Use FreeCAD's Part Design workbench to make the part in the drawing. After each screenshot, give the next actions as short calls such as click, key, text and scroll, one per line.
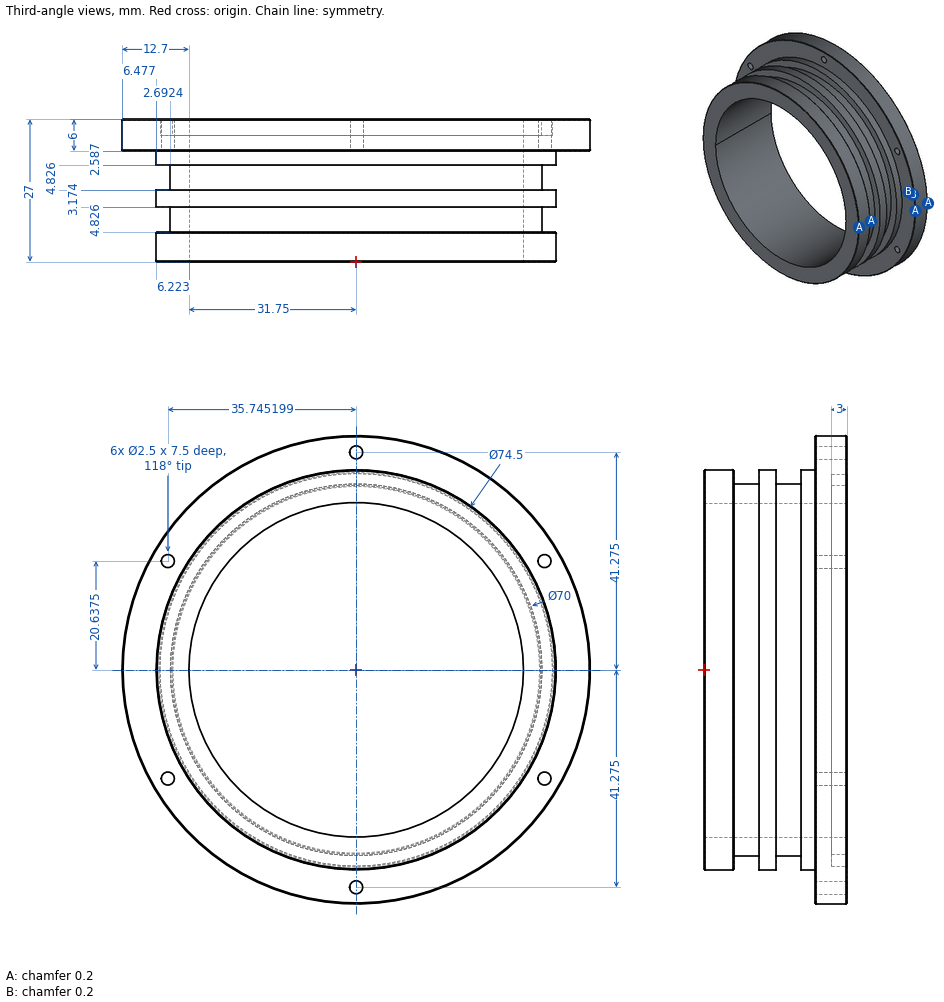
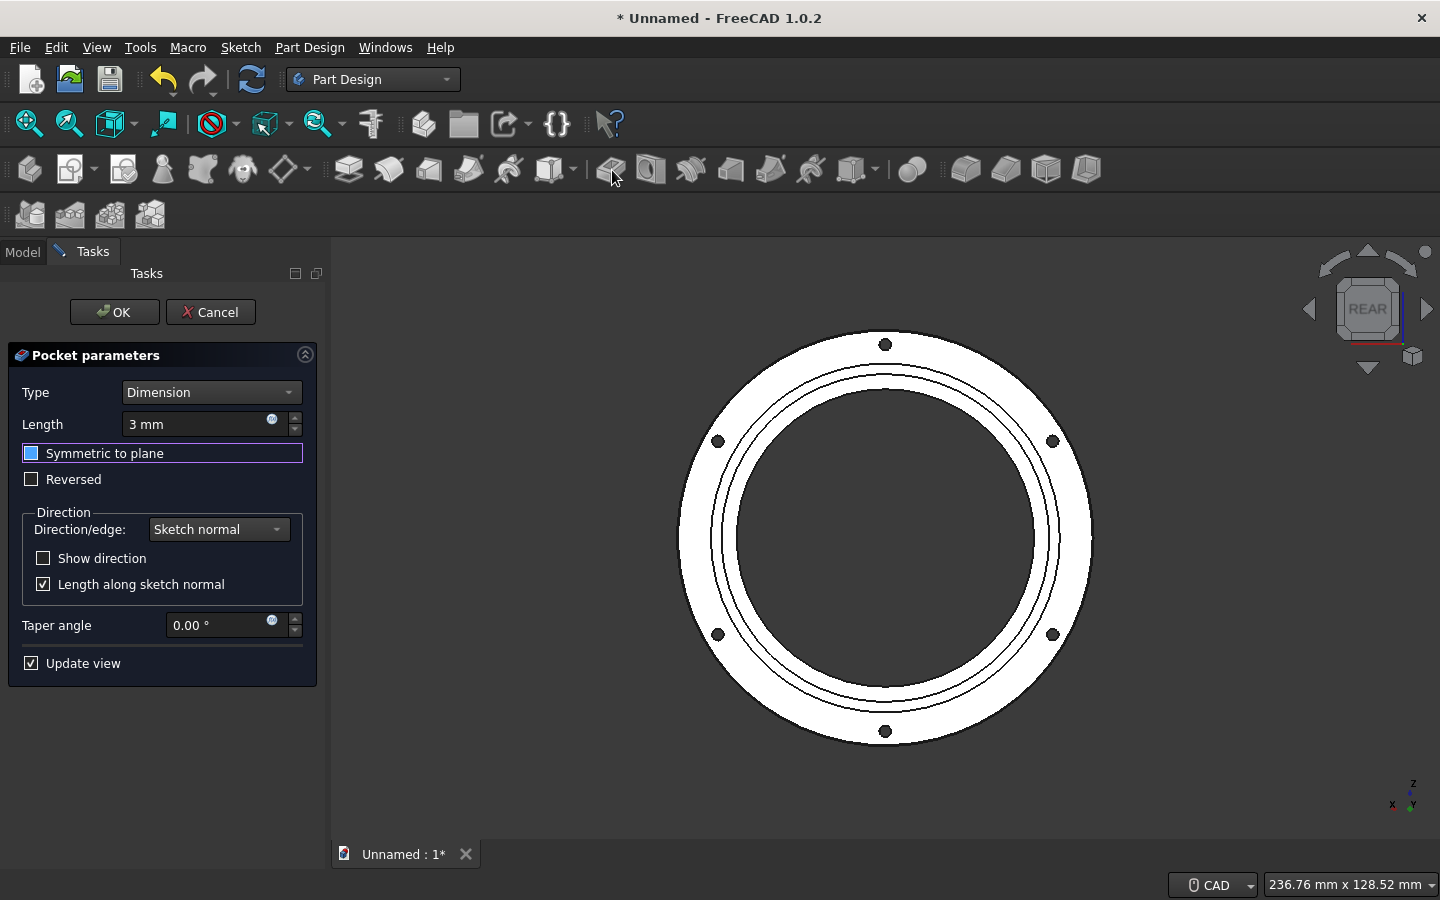
click(115, 312)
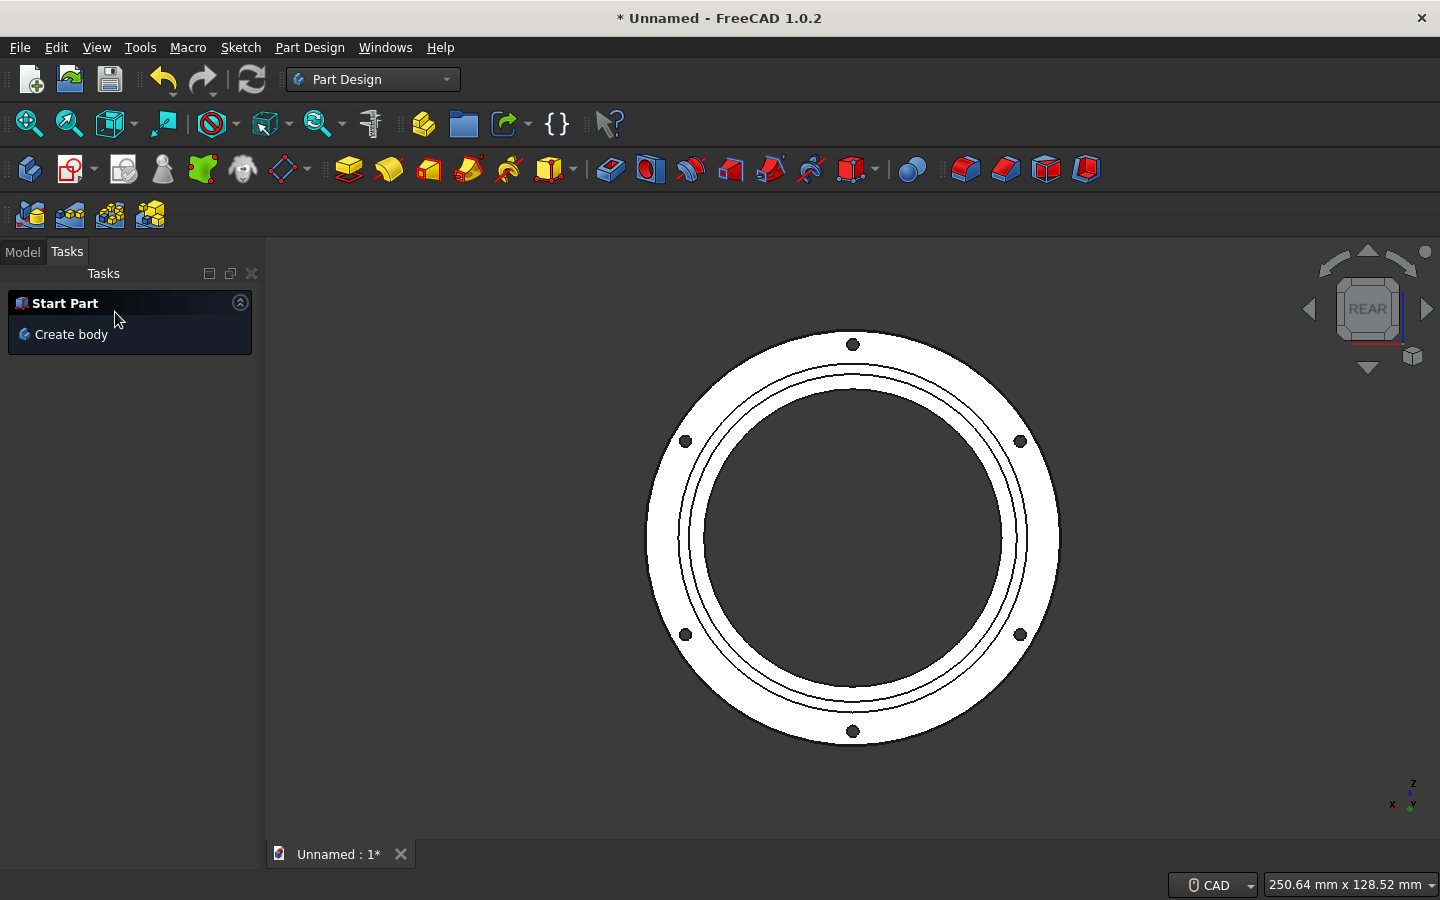
click(678, 537)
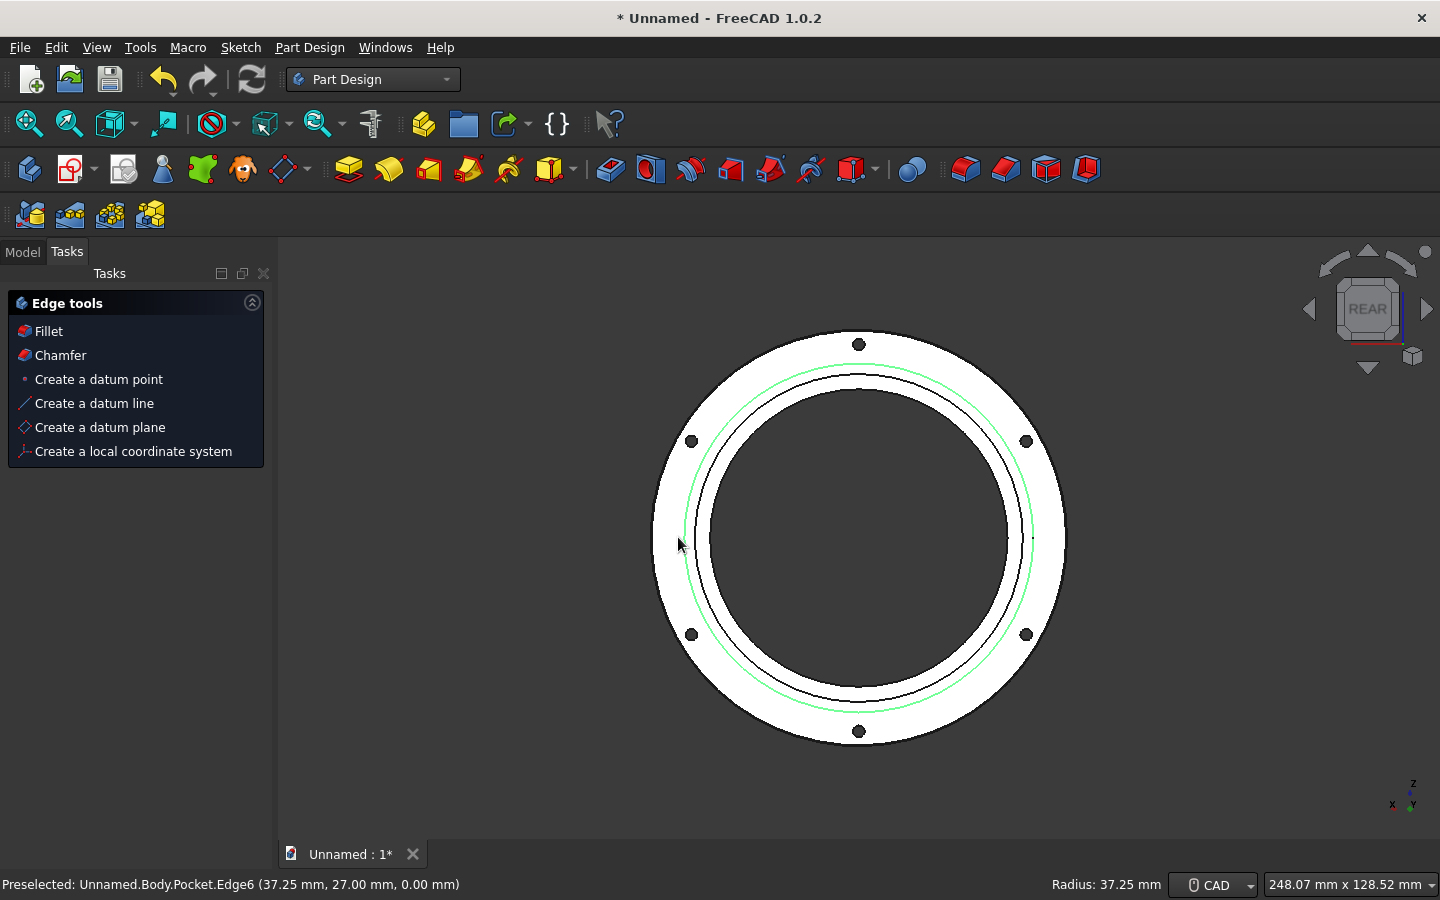
click(910, 381, ctrl)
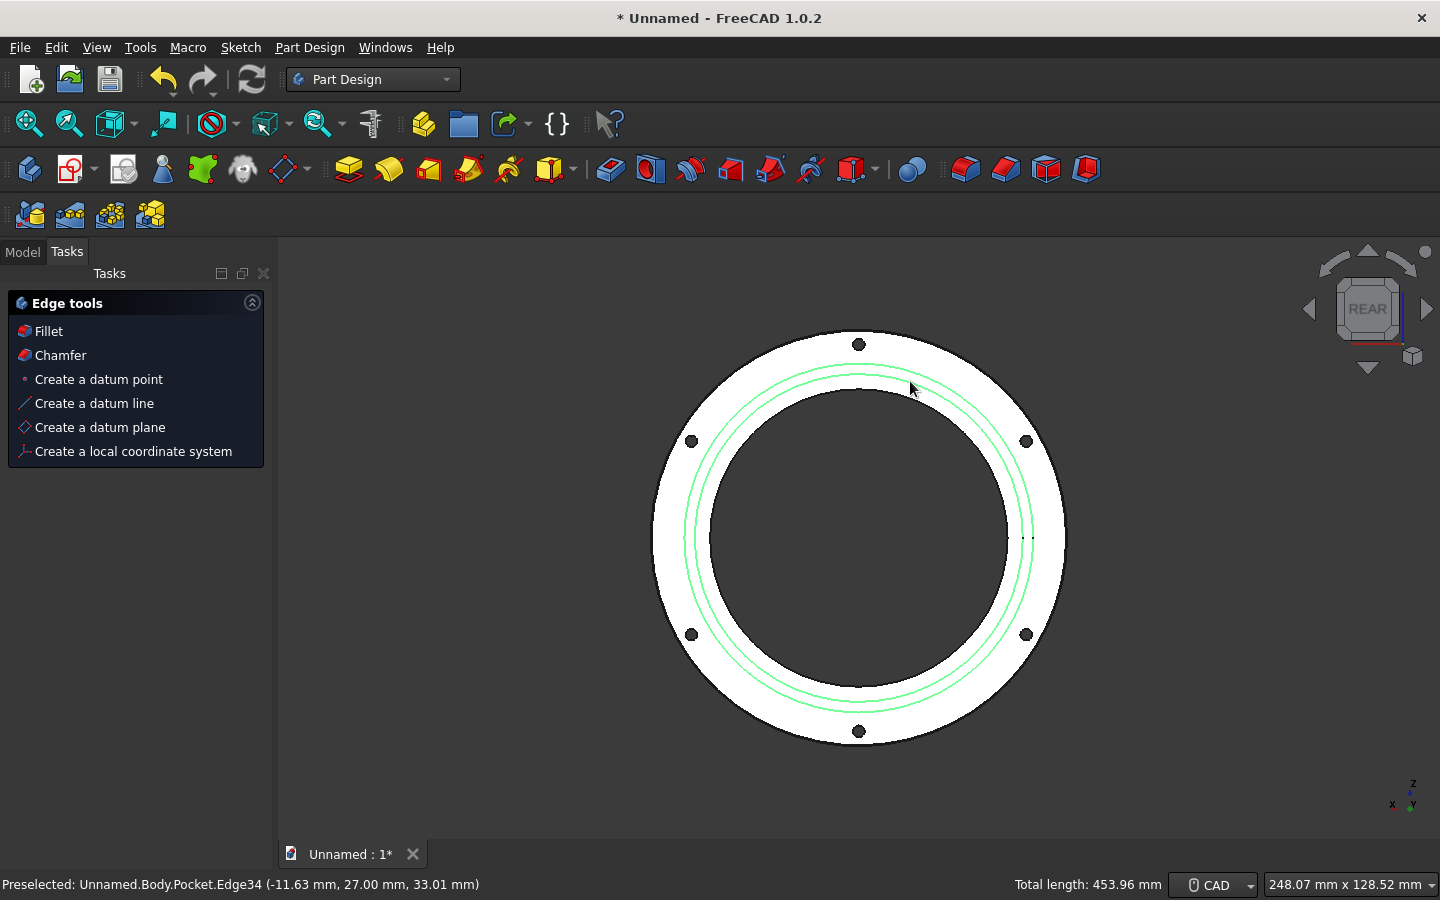
click(1006, 170)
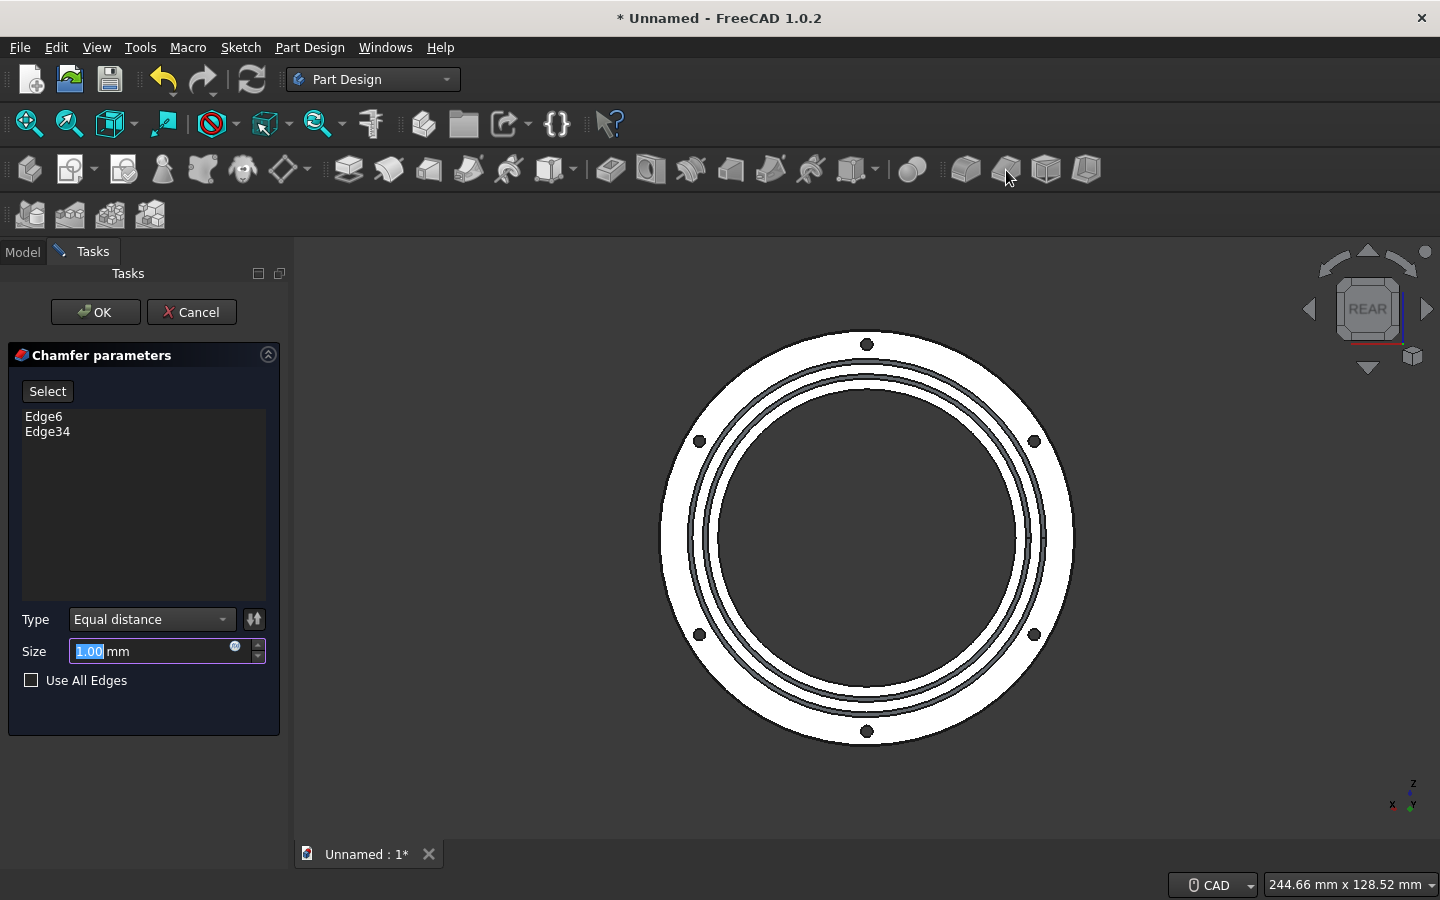
text(0.2)
key(Tab)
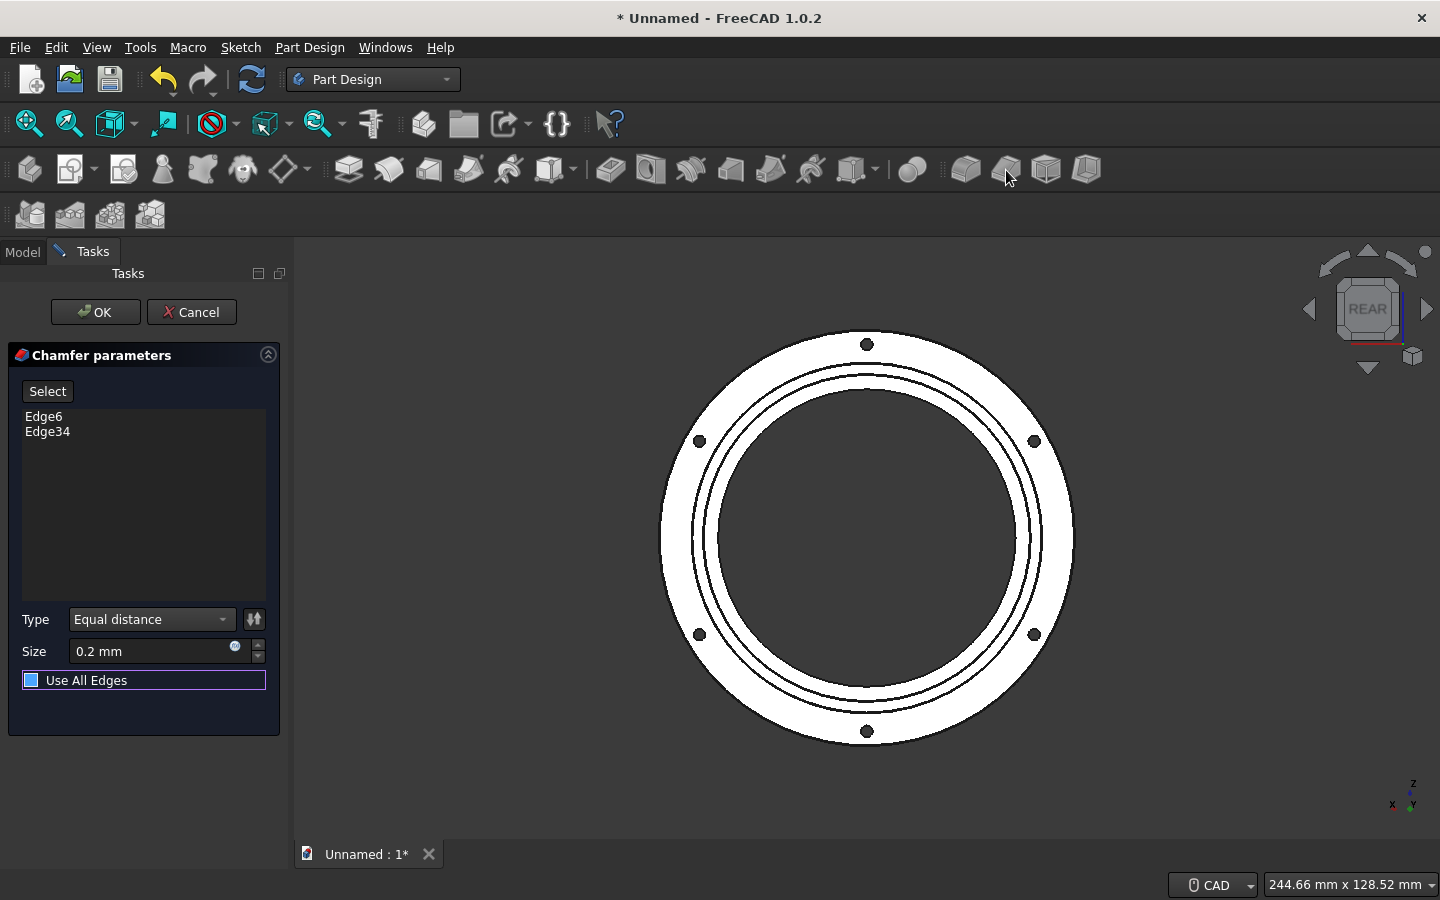
click(96, 312)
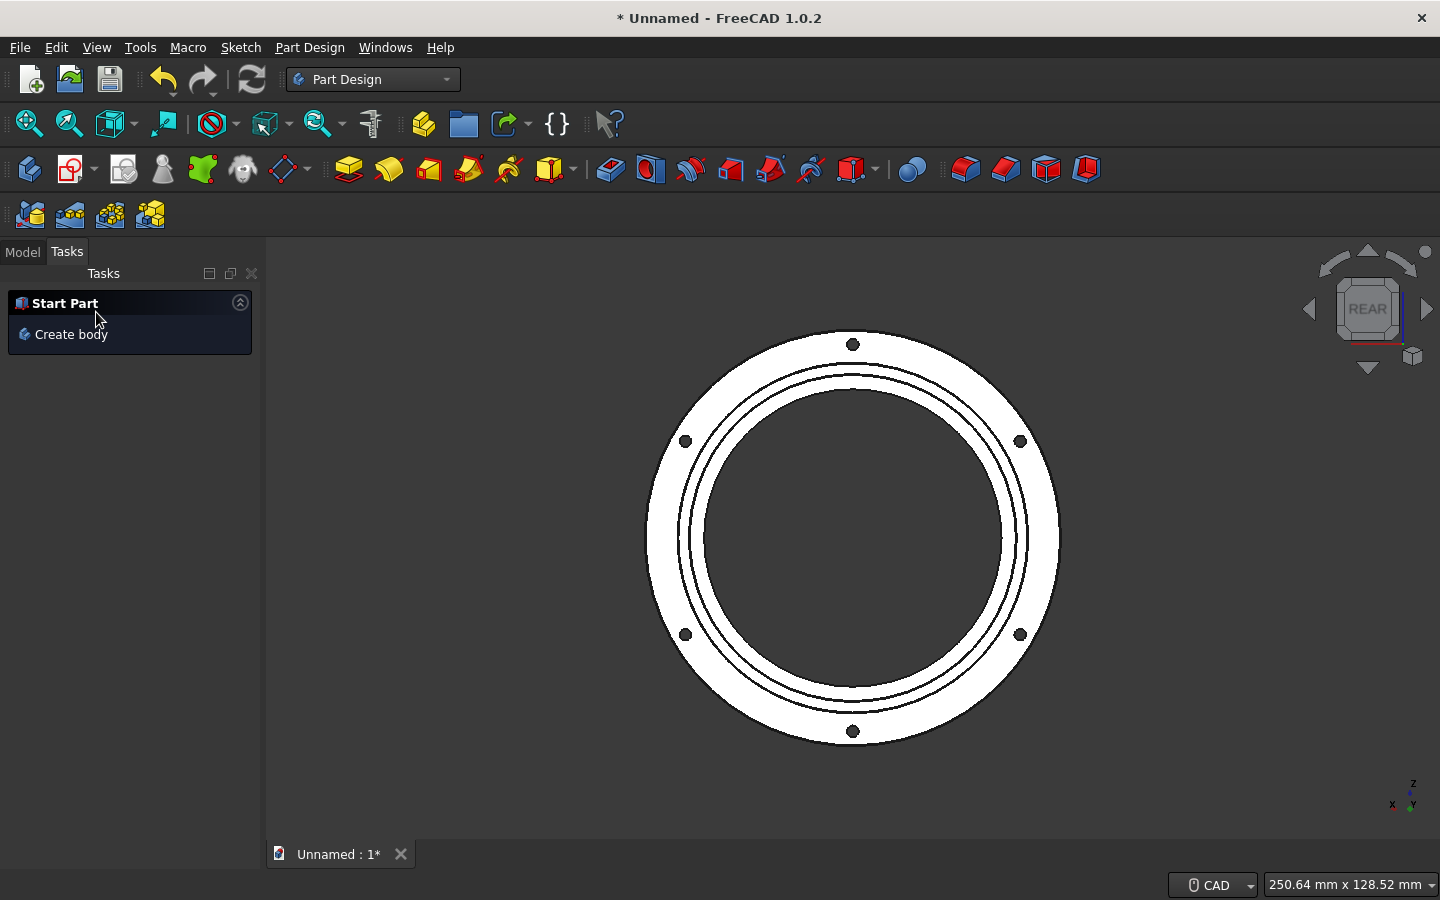
key(0)